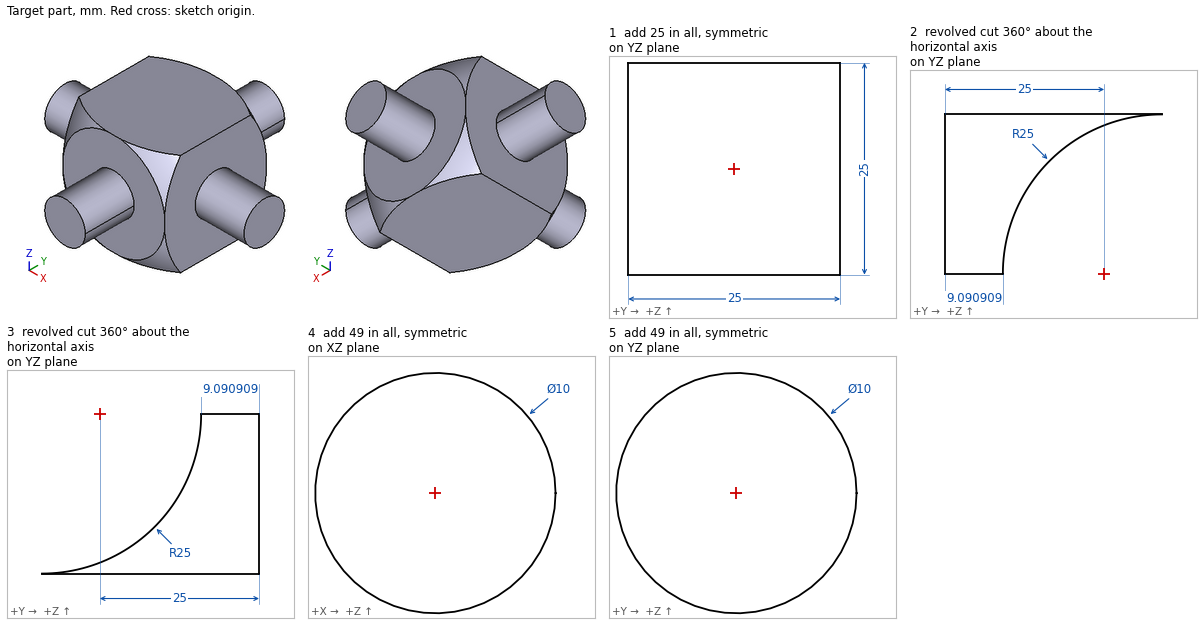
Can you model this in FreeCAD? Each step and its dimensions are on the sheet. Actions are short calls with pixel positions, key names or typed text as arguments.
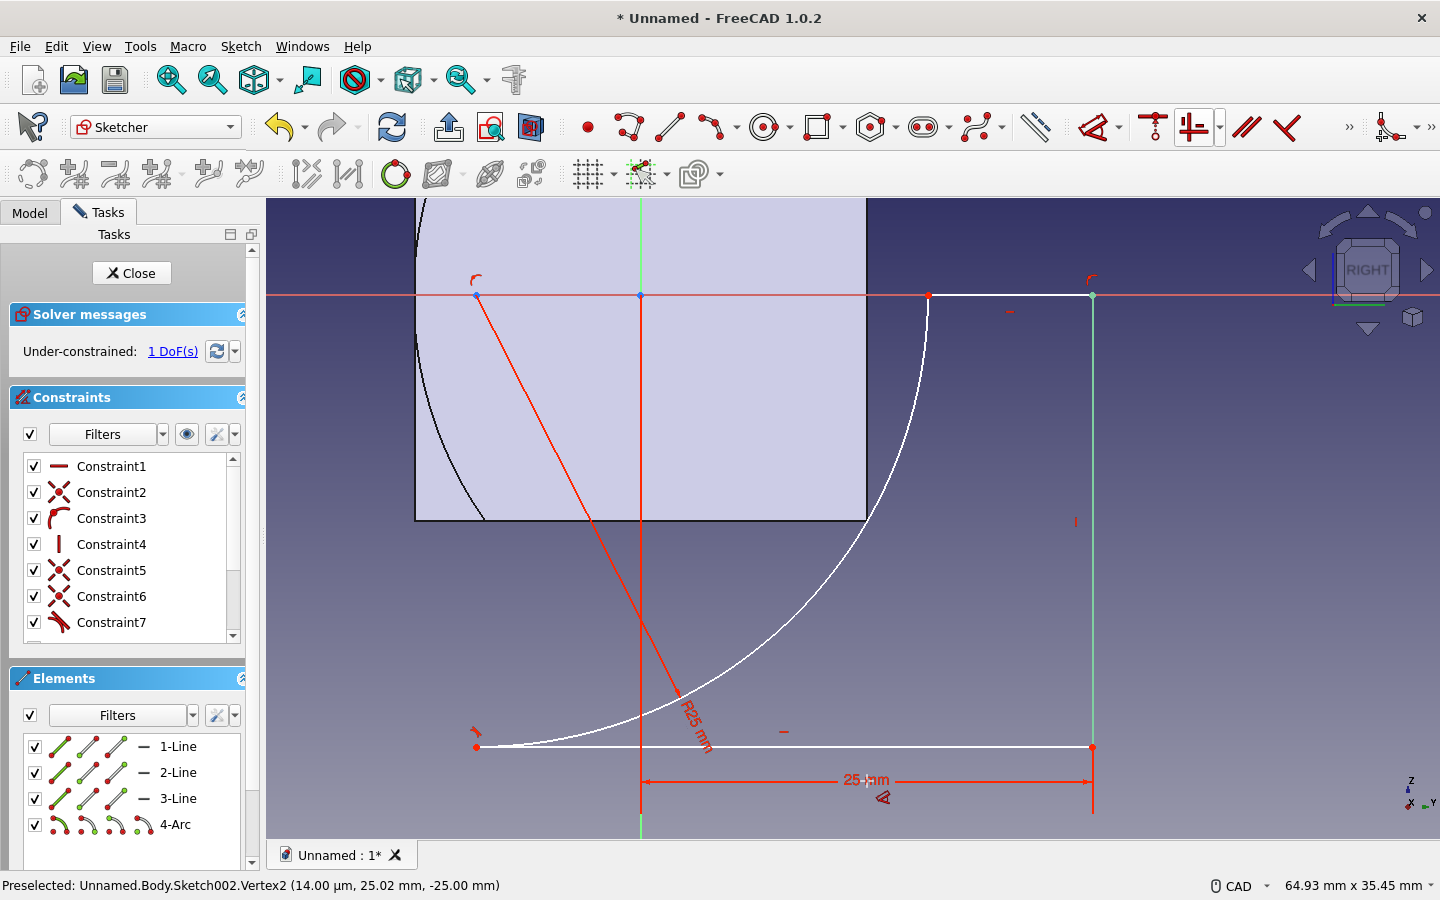
click(1043, 295)
click(1010, 261)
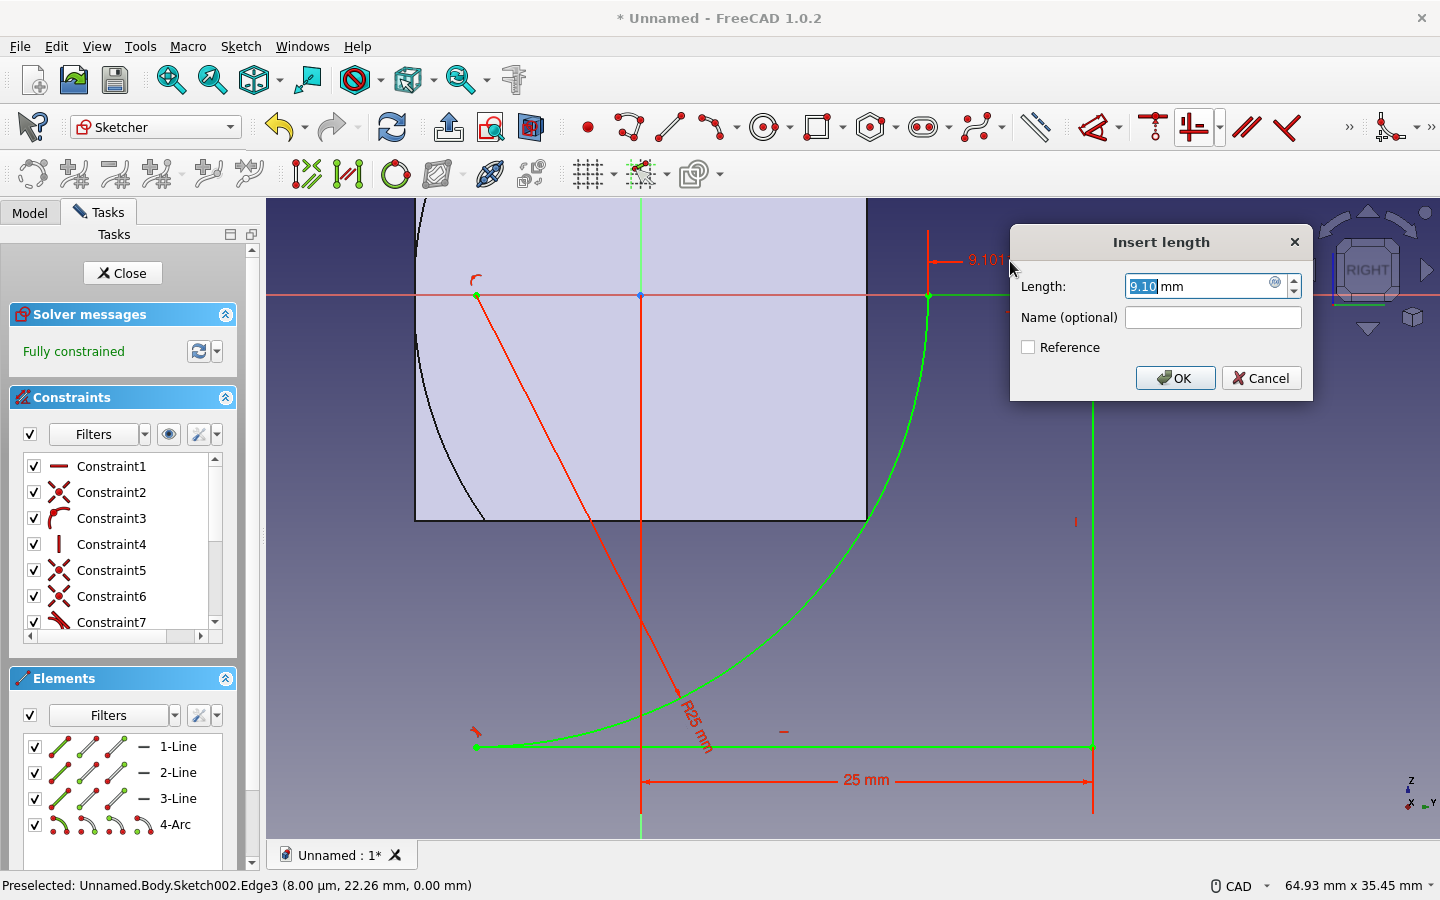
text(9.090909)
key(Return)
key(Escape)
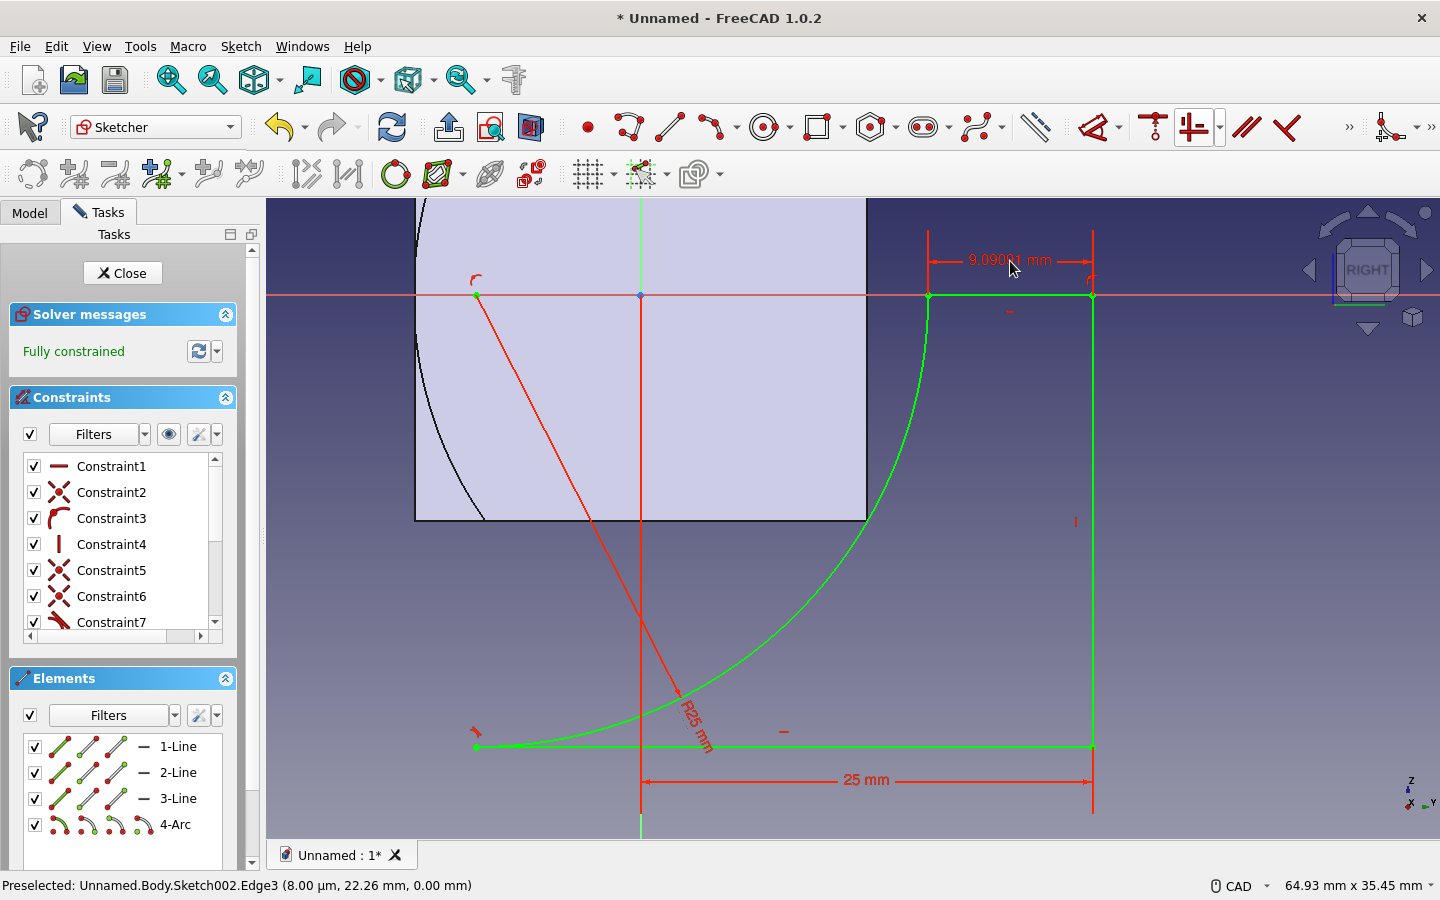
click(123, 273)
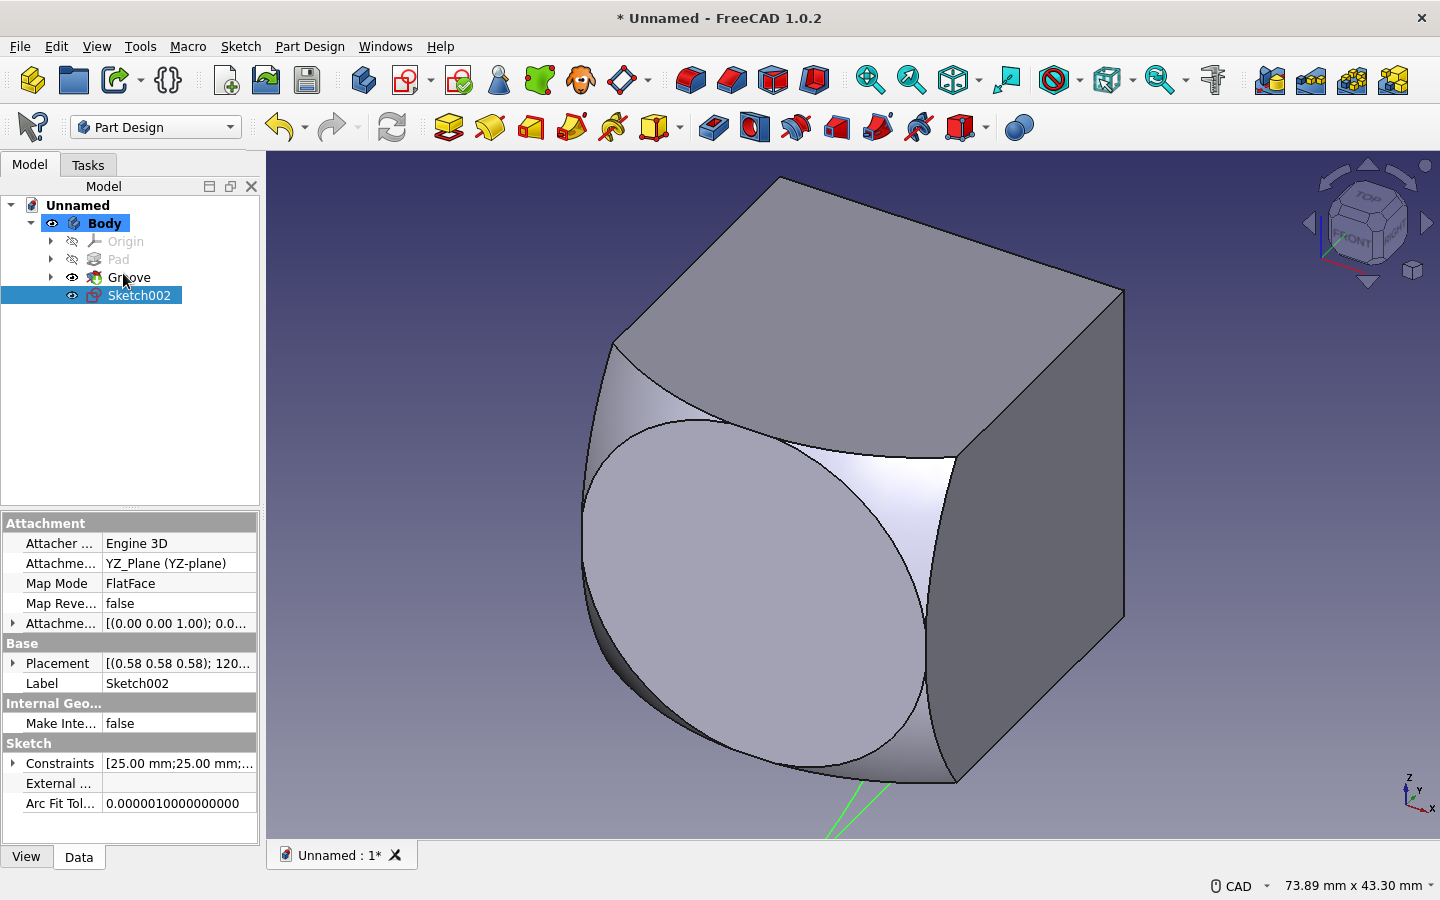
click(796, 128)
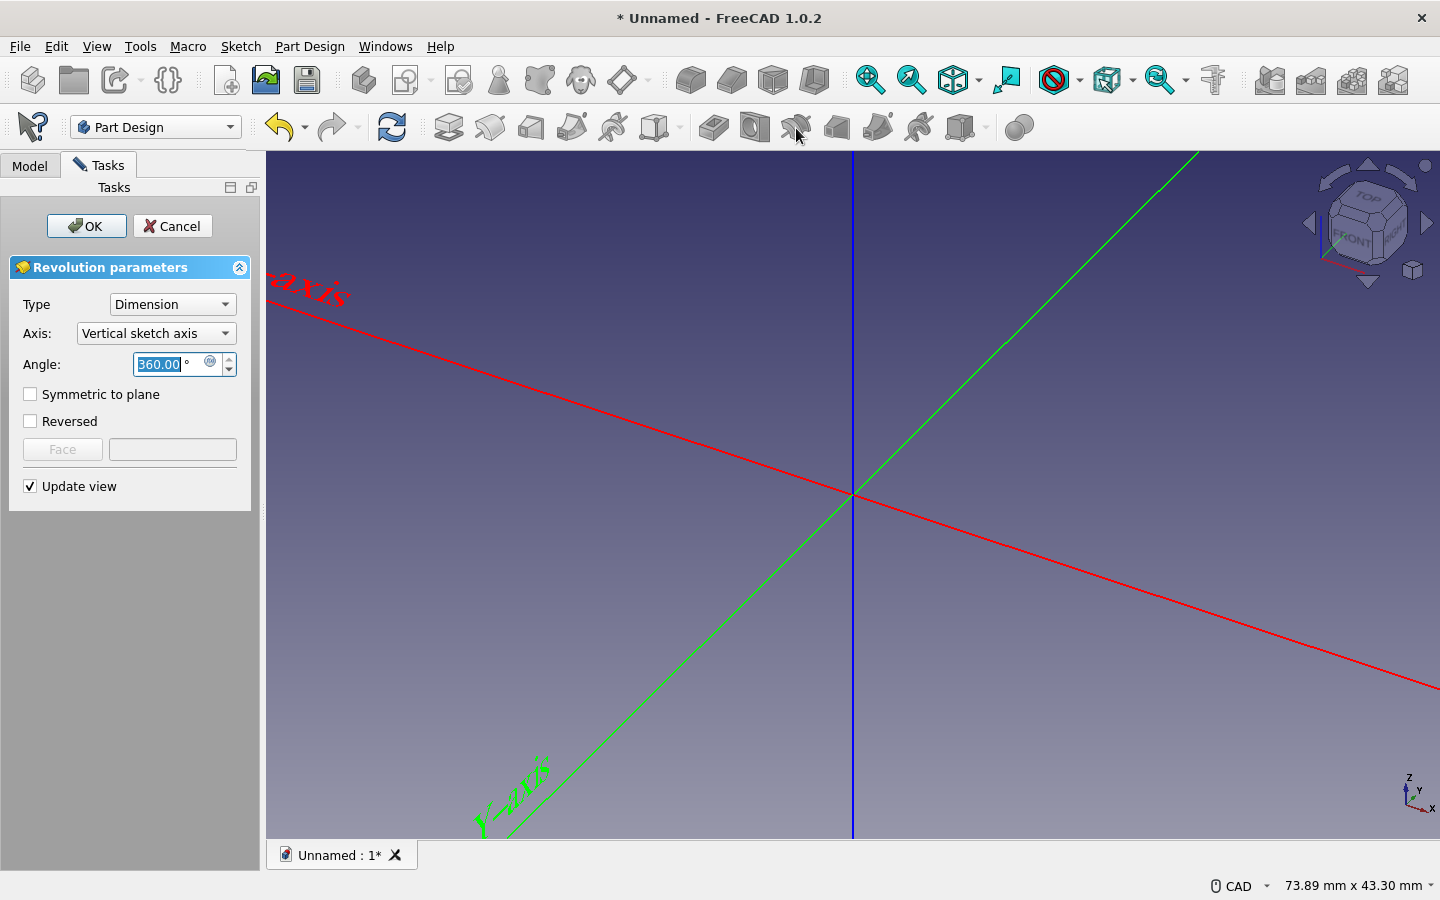
click(157, 334)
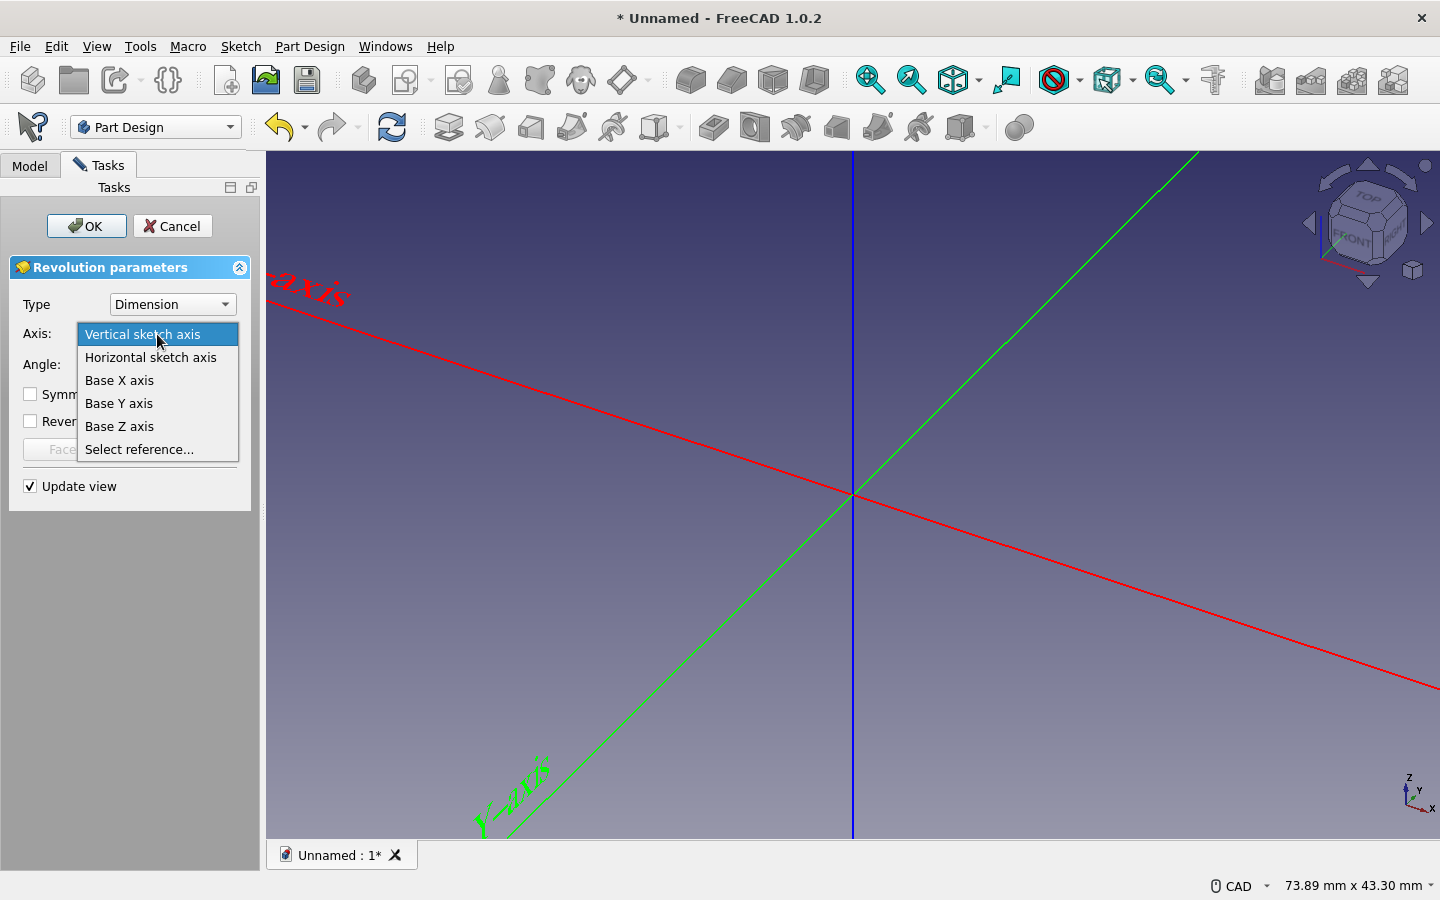
click(156, 358)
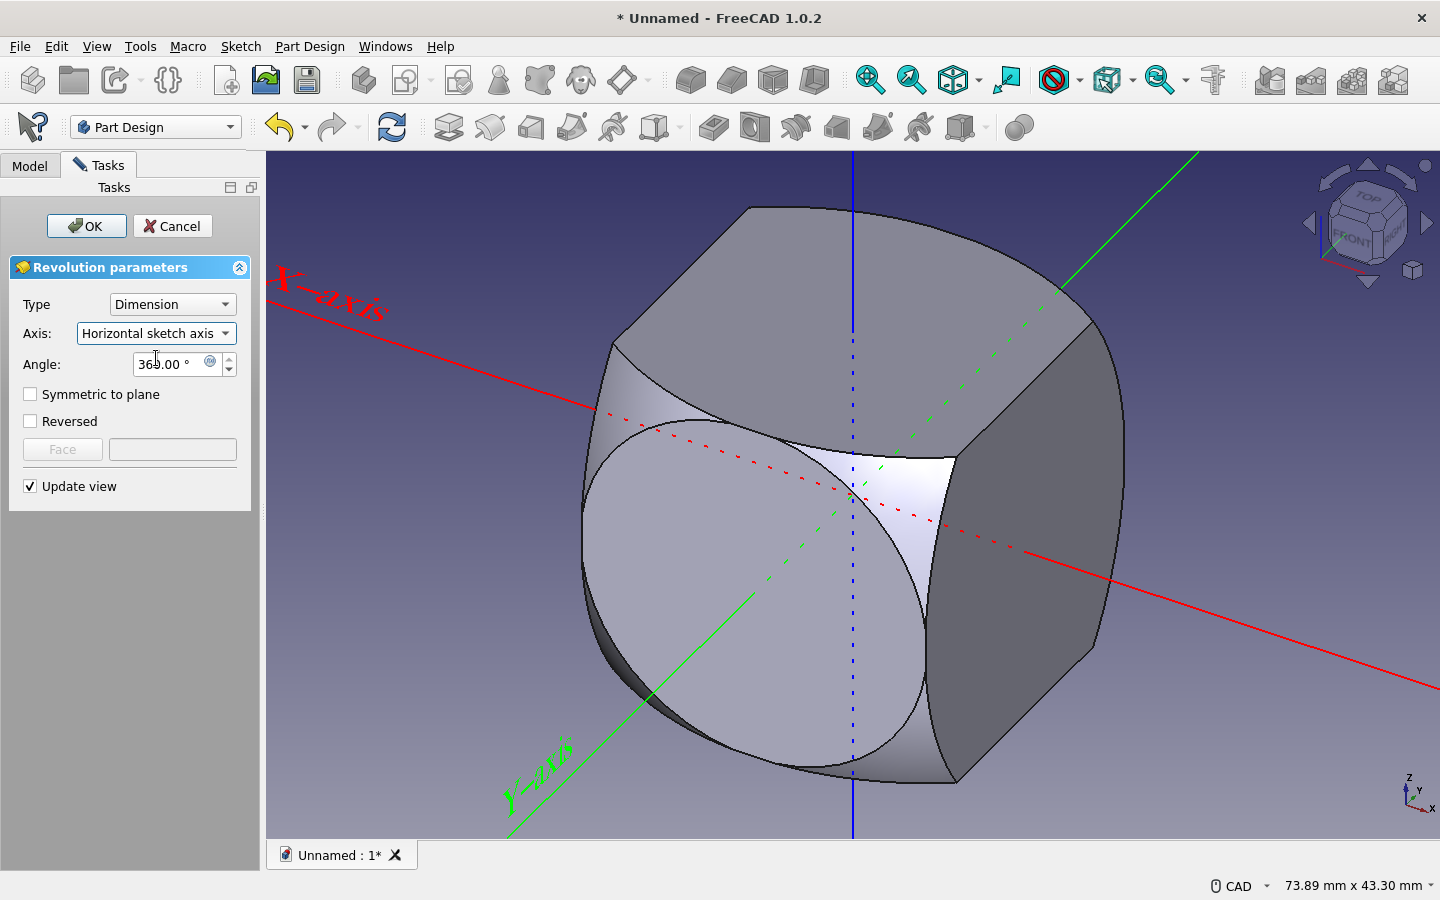
click(87, 226)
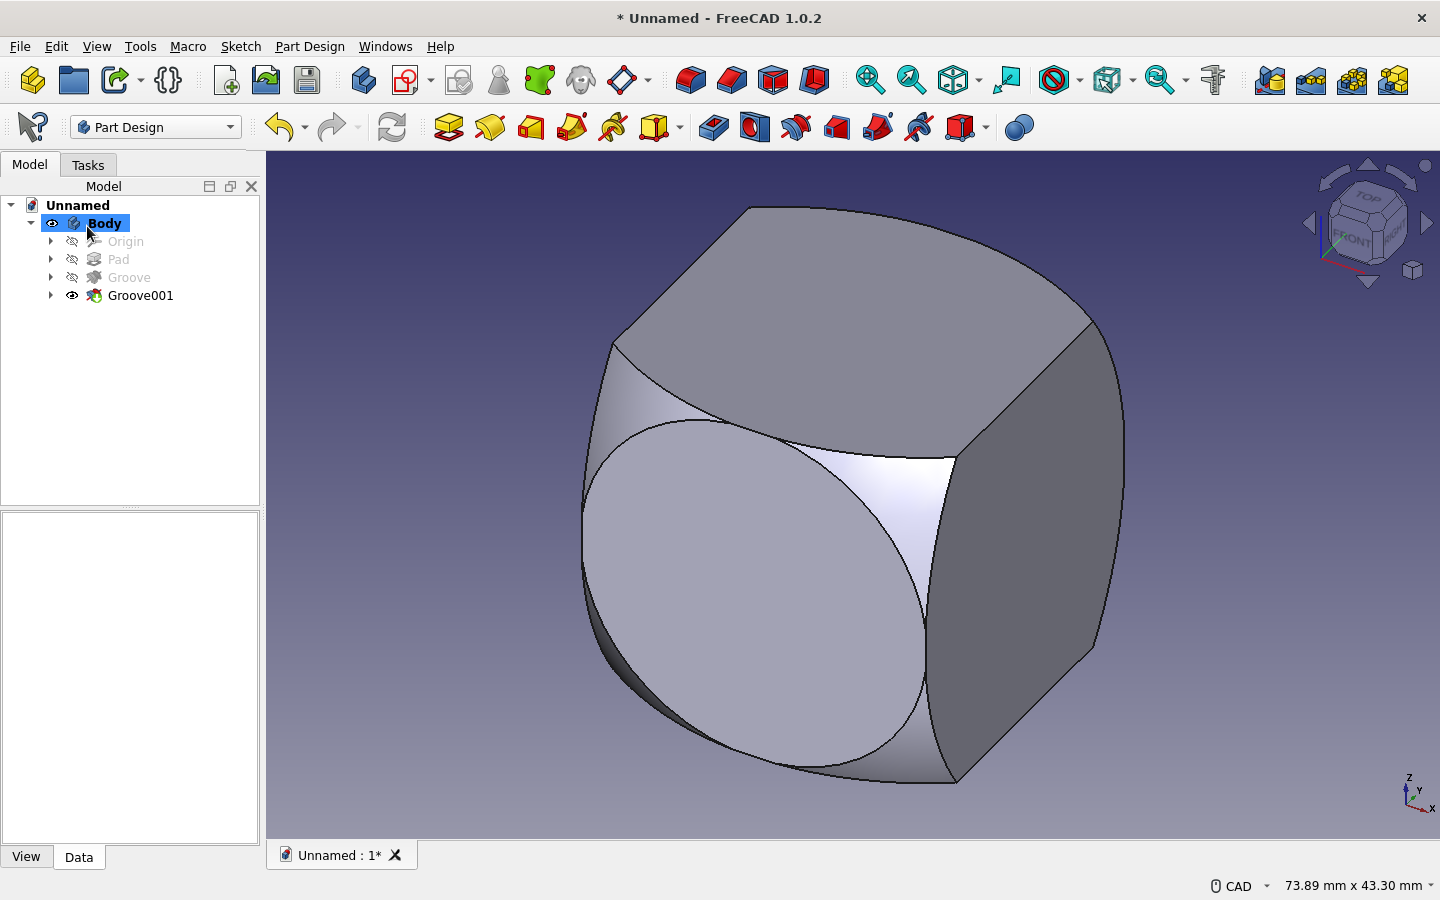
click(404, 80)